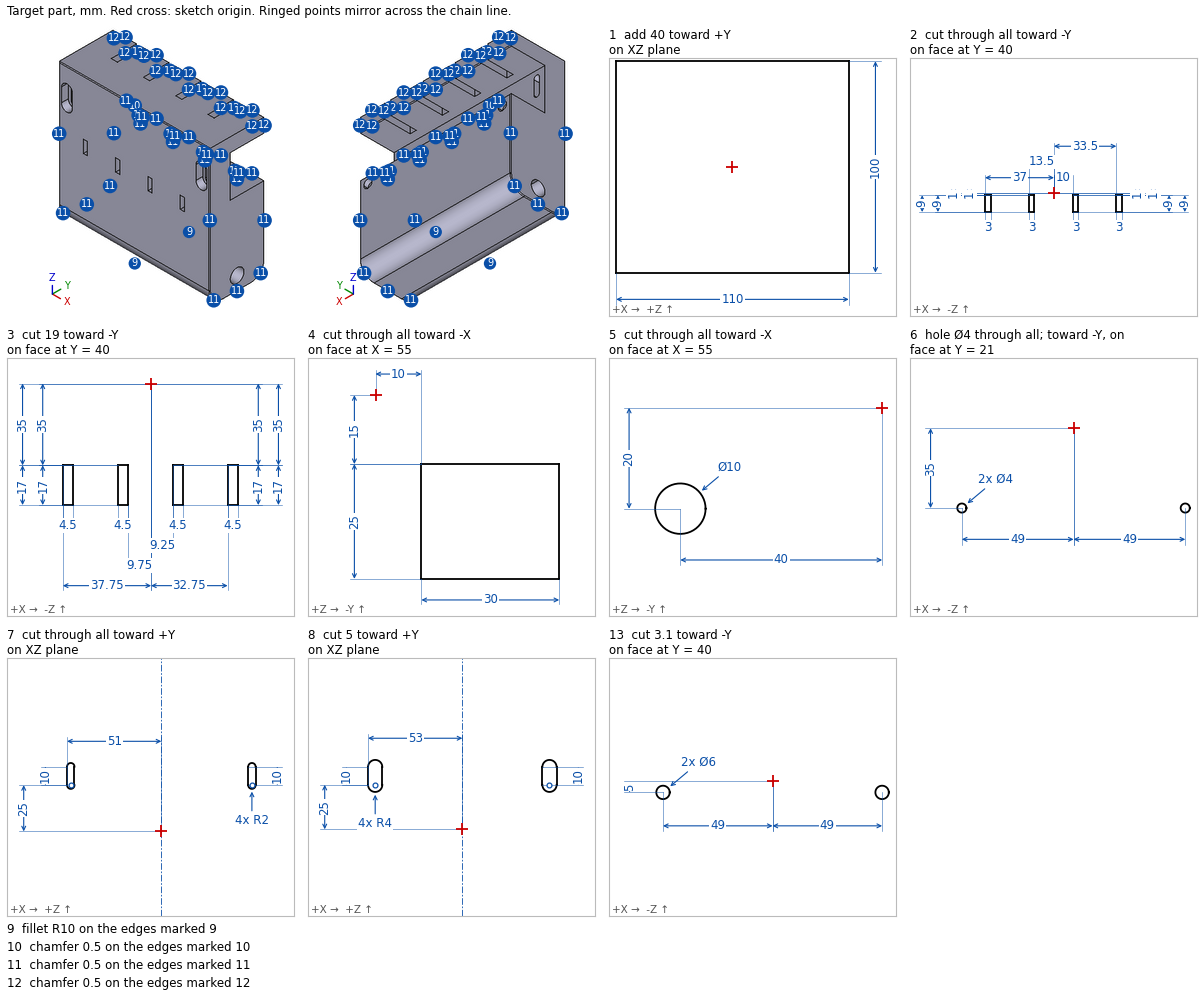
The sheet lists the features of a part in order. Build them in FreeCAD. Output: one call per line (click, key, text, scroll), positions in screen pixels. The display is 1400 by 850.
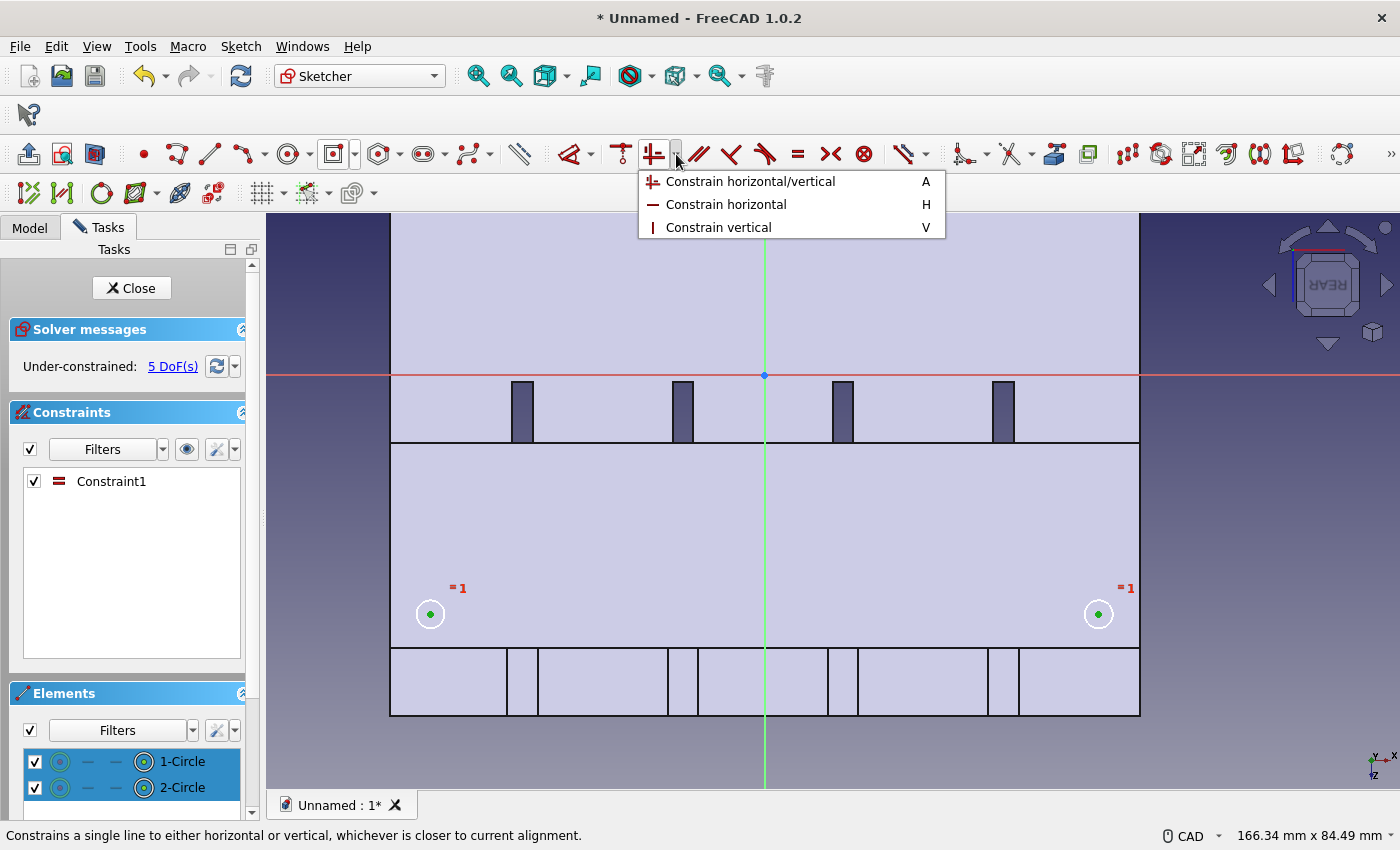
click(792, 204)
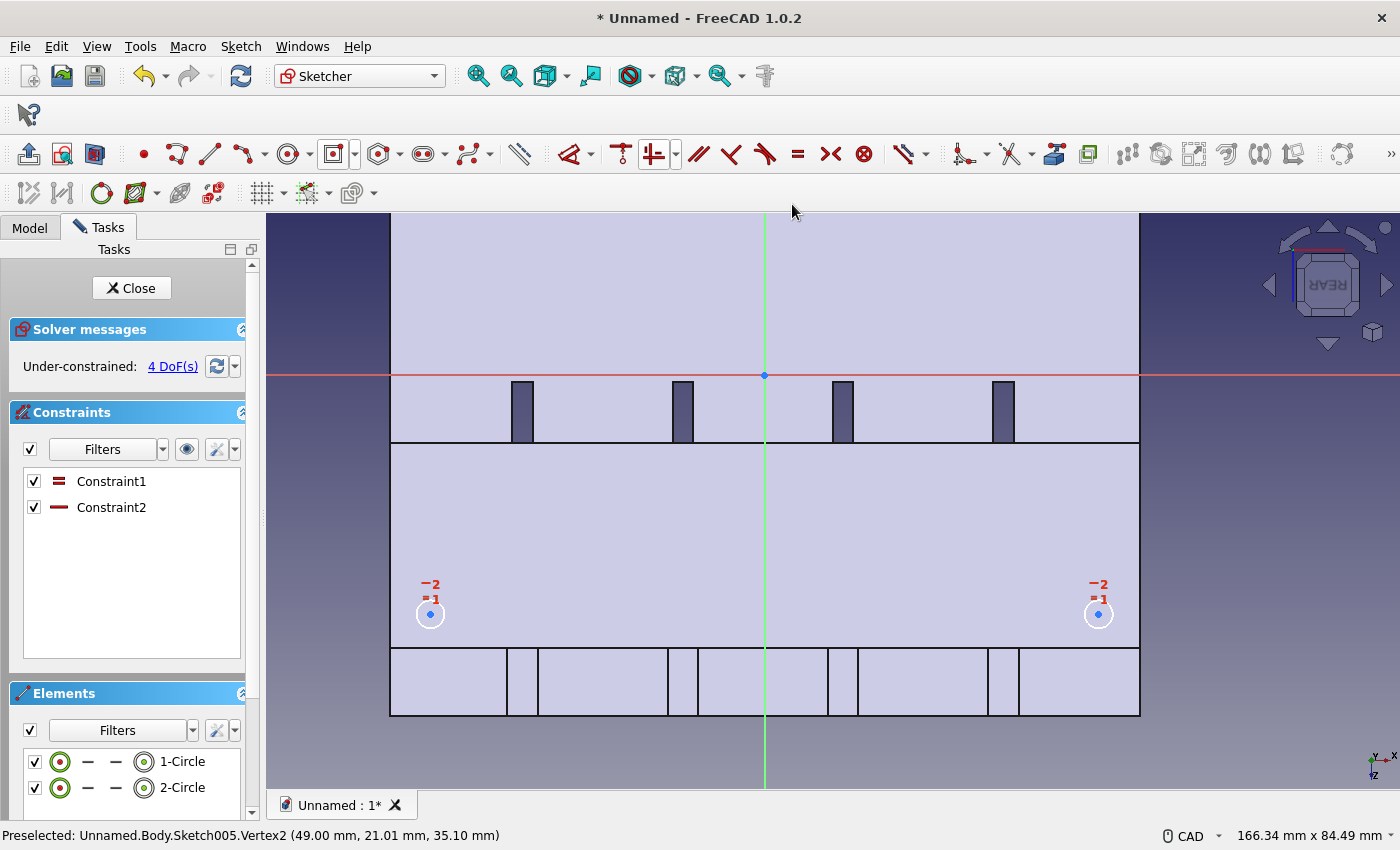
click(568, 154)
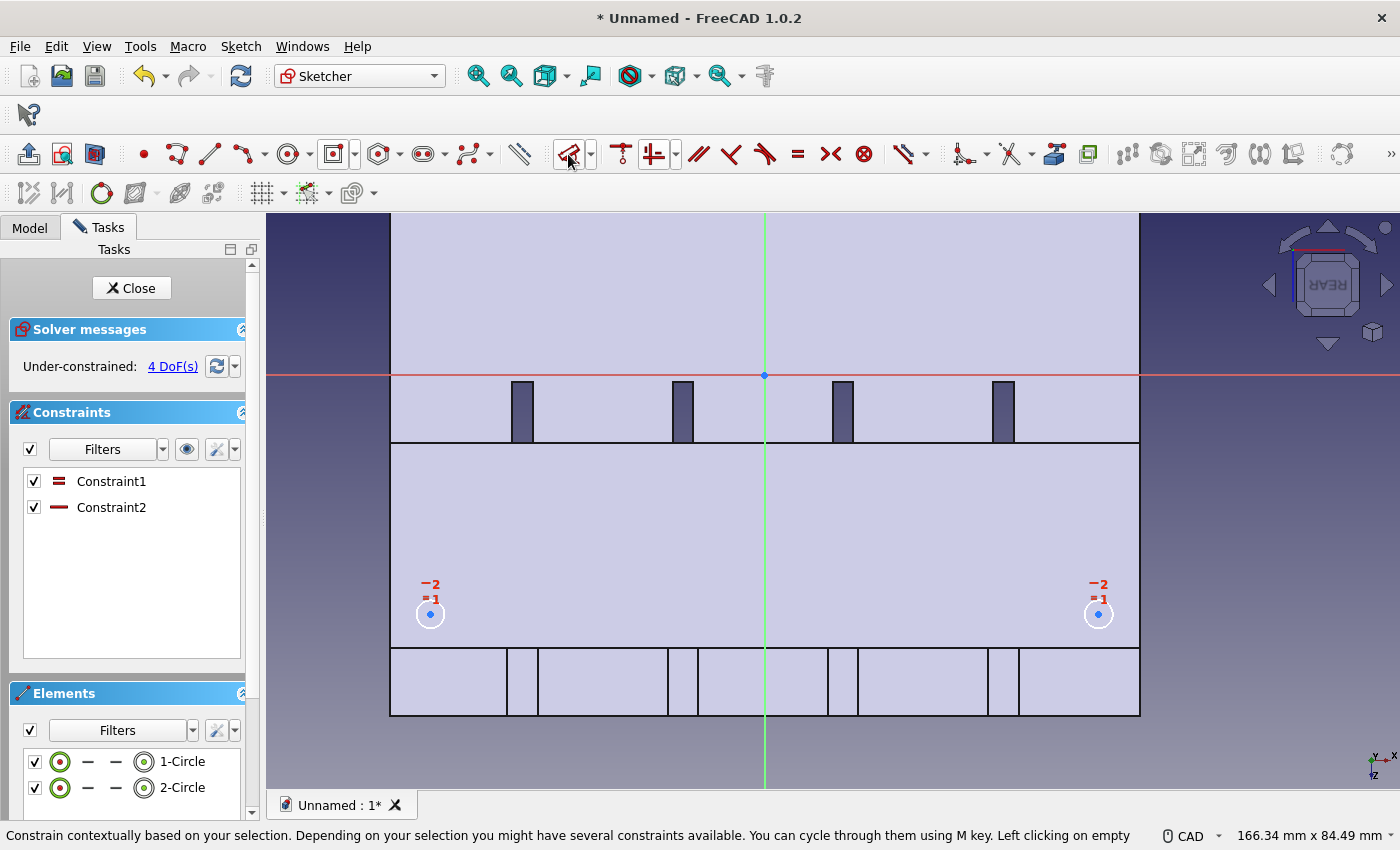
scroll(440, 604, up, 2)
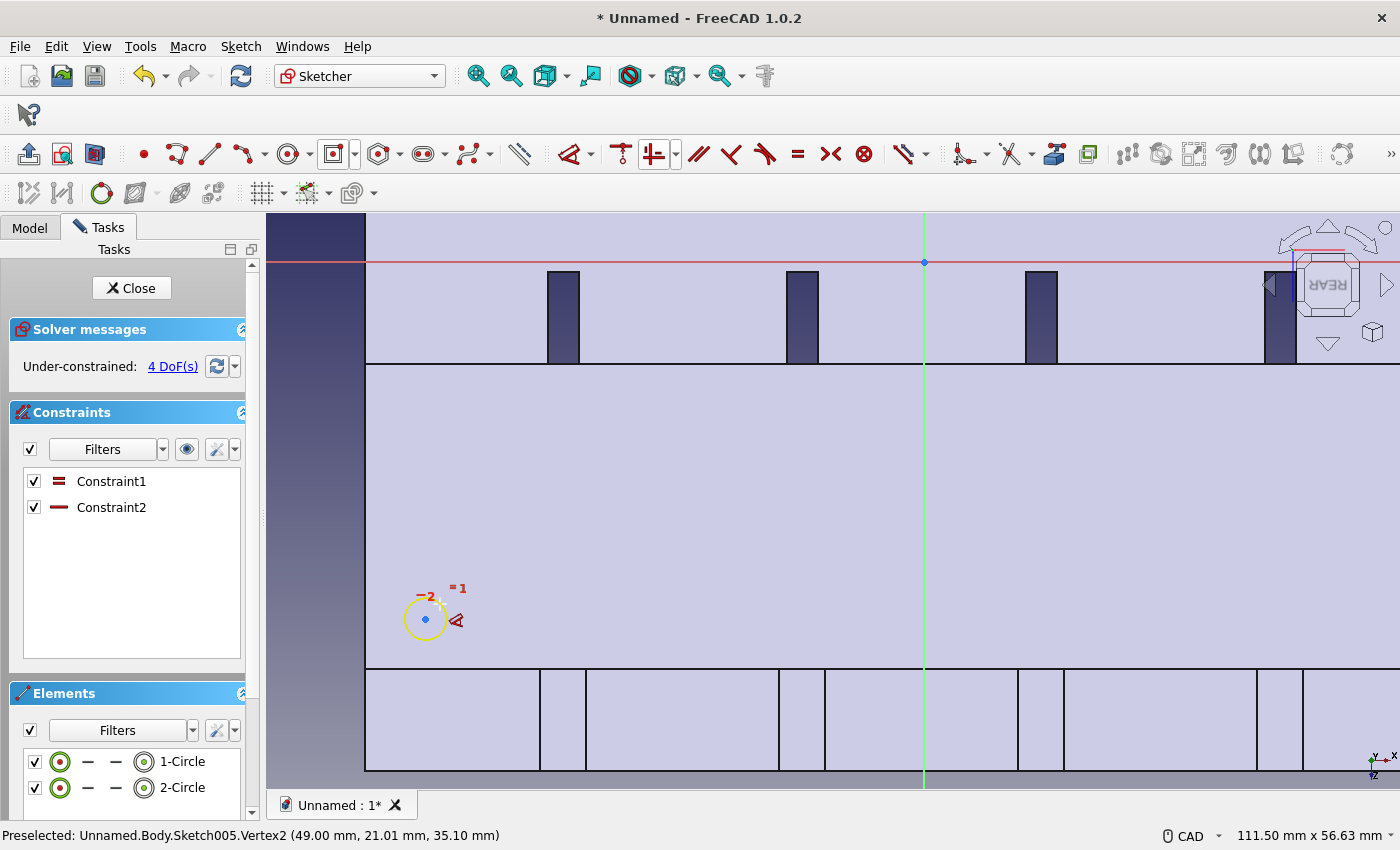
click(440, 604)
click(462, 581)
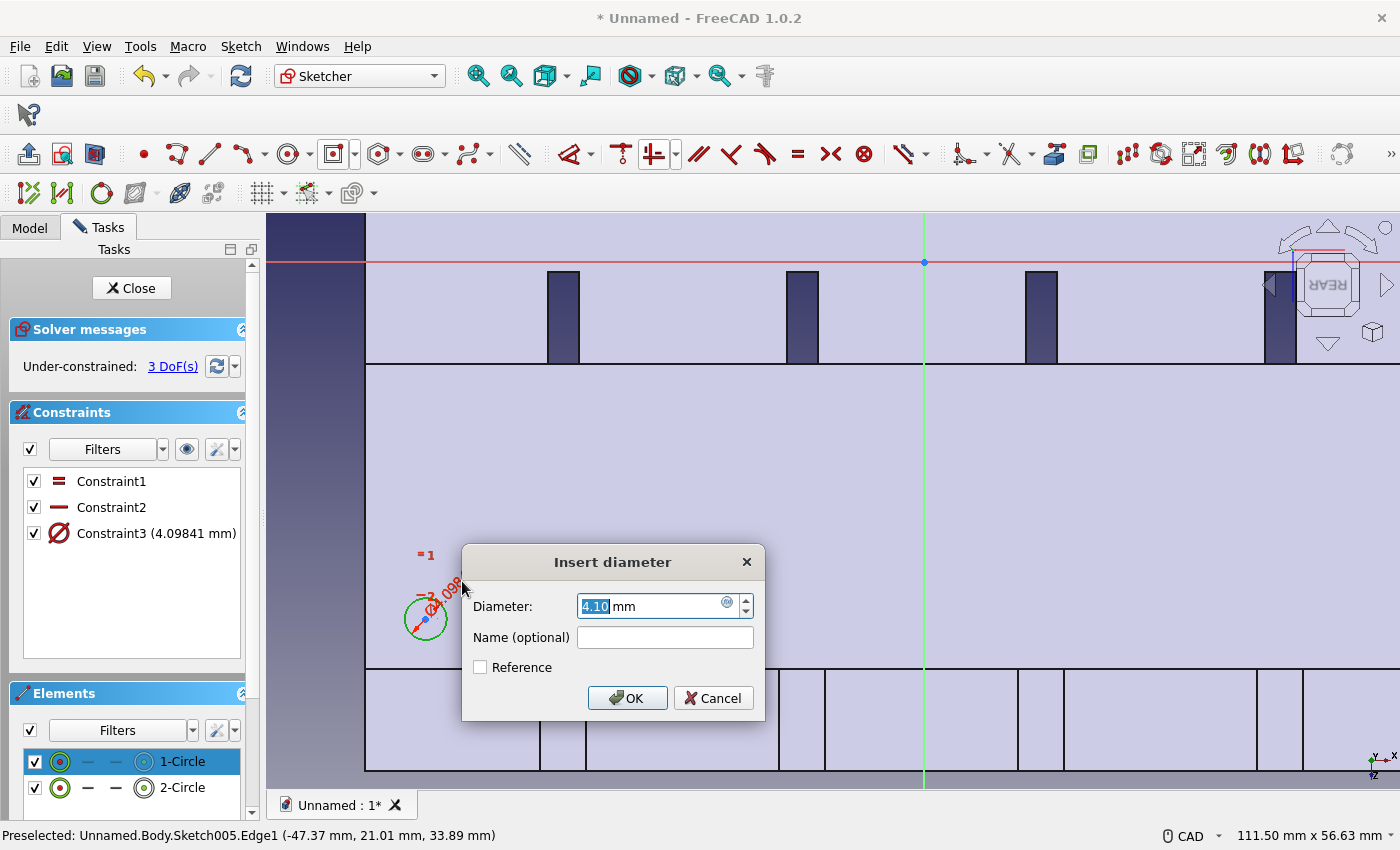
text(4)
key(Return)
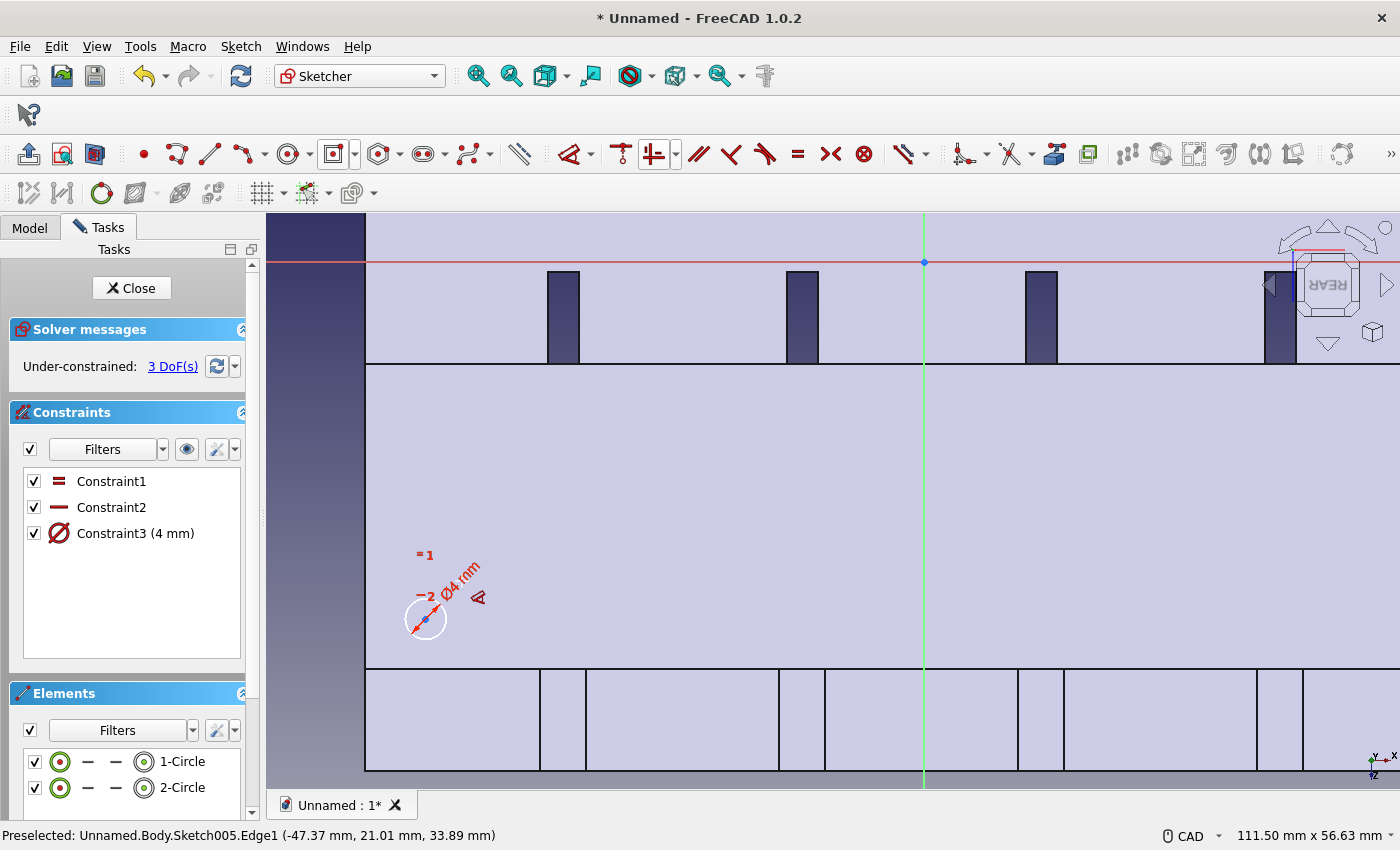
click(426, 619)
click(675, 653)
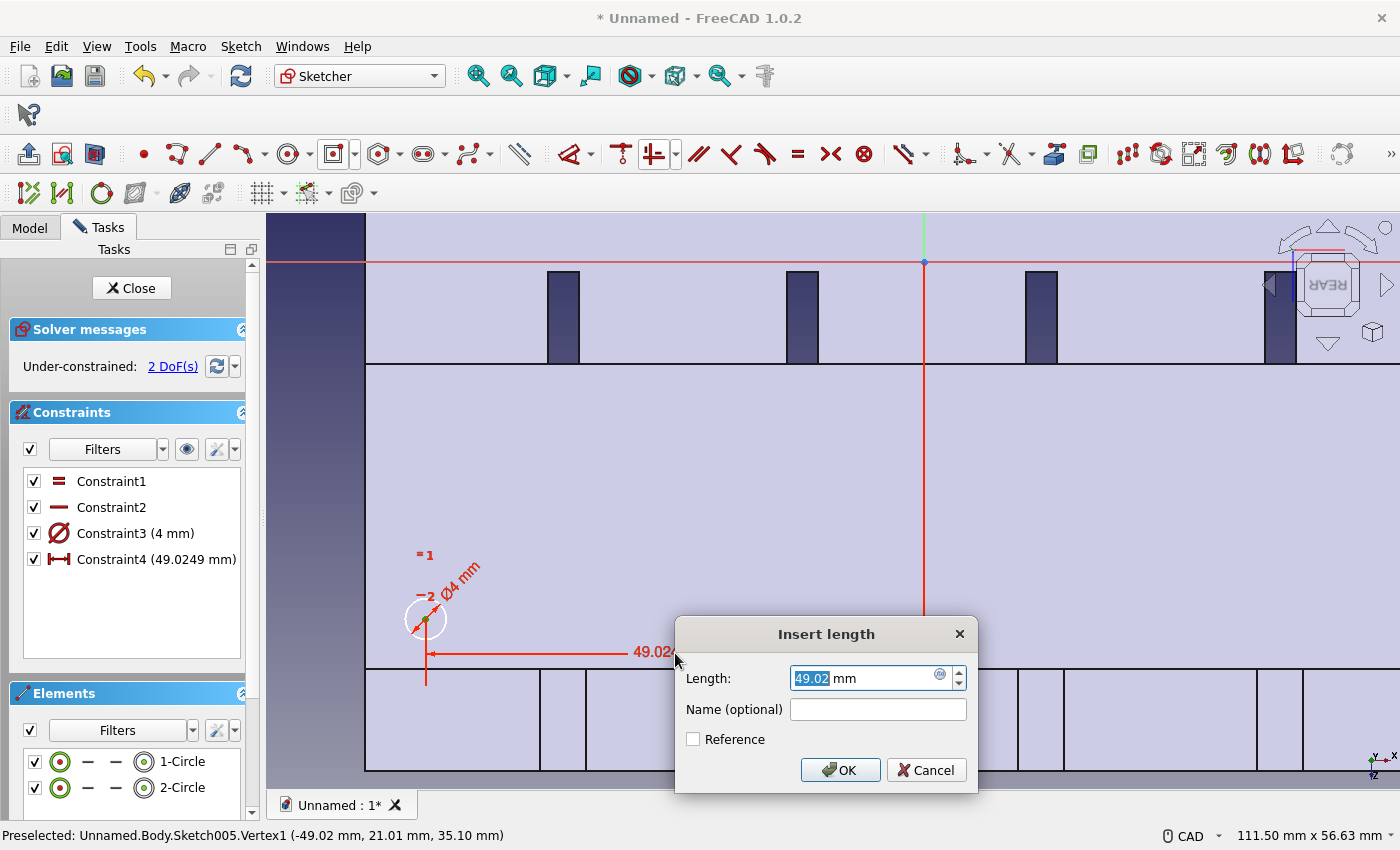
text(49)
key(Return)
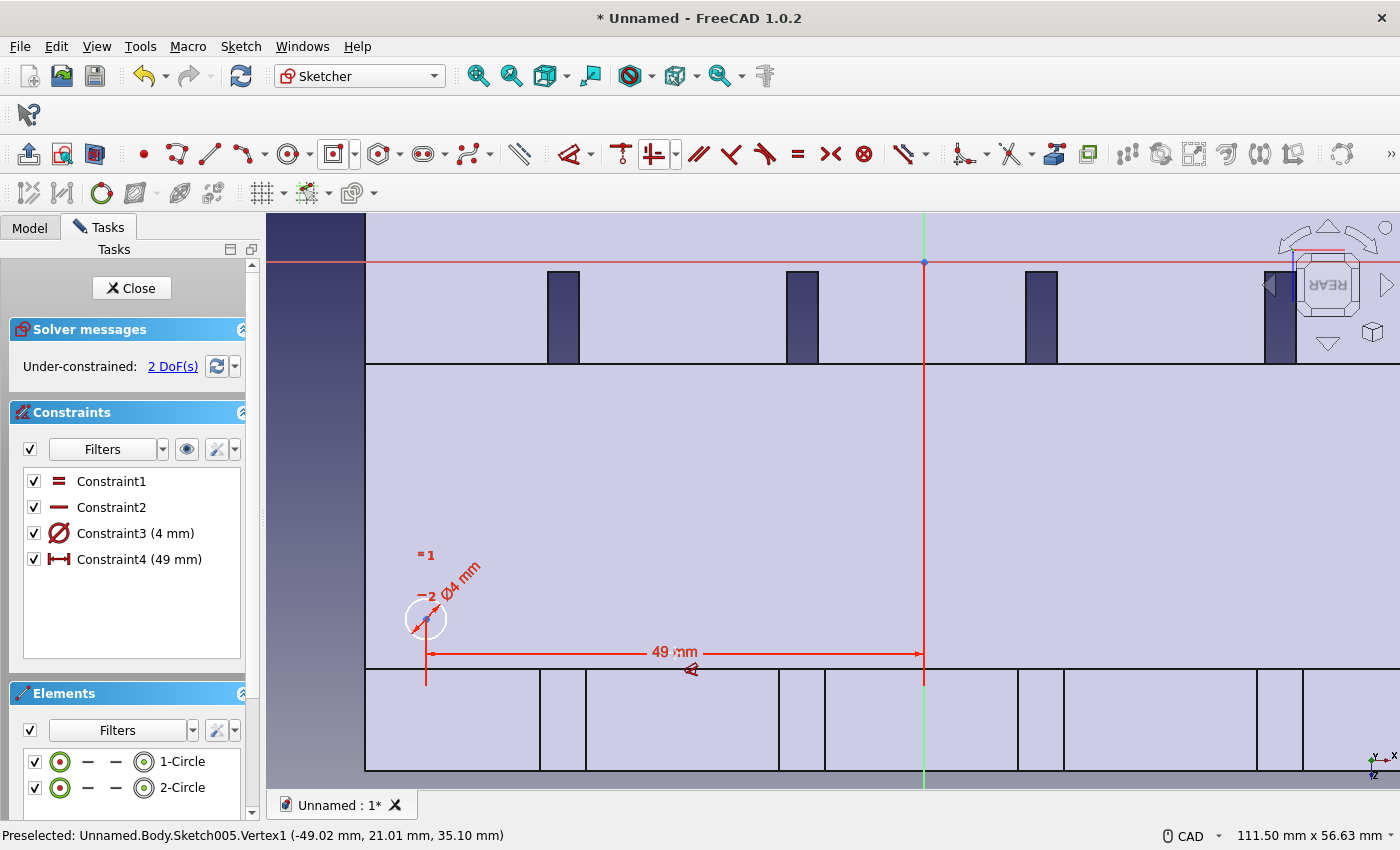
click(426, 619)
click(392, 441)